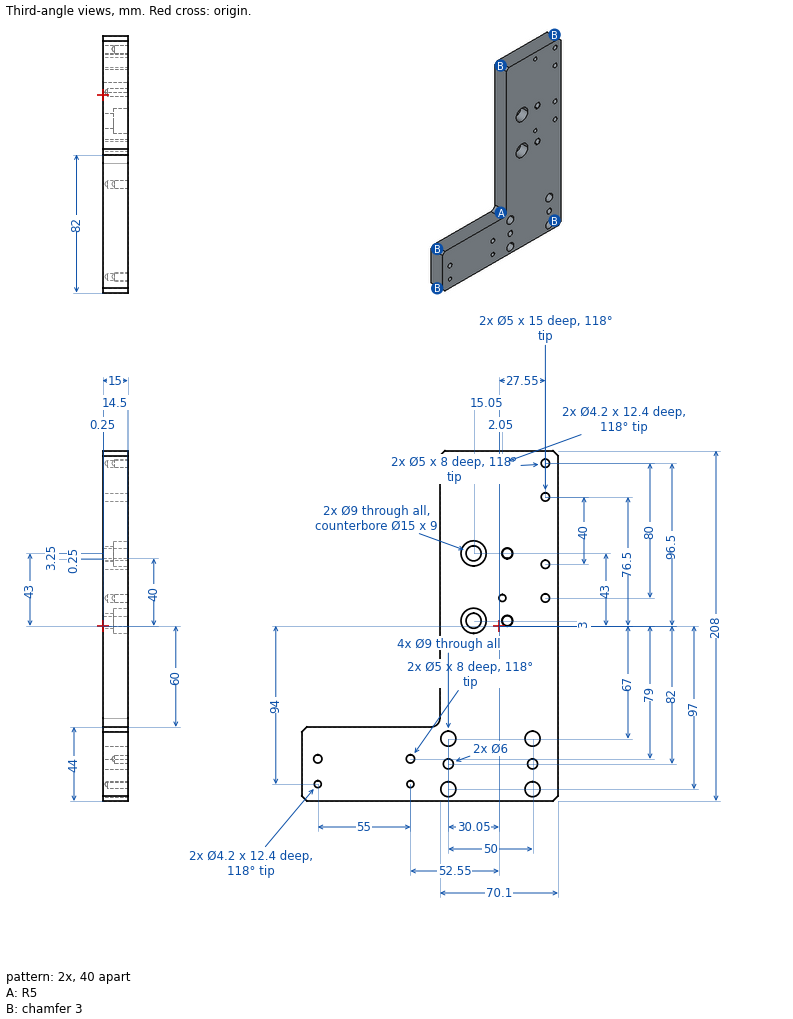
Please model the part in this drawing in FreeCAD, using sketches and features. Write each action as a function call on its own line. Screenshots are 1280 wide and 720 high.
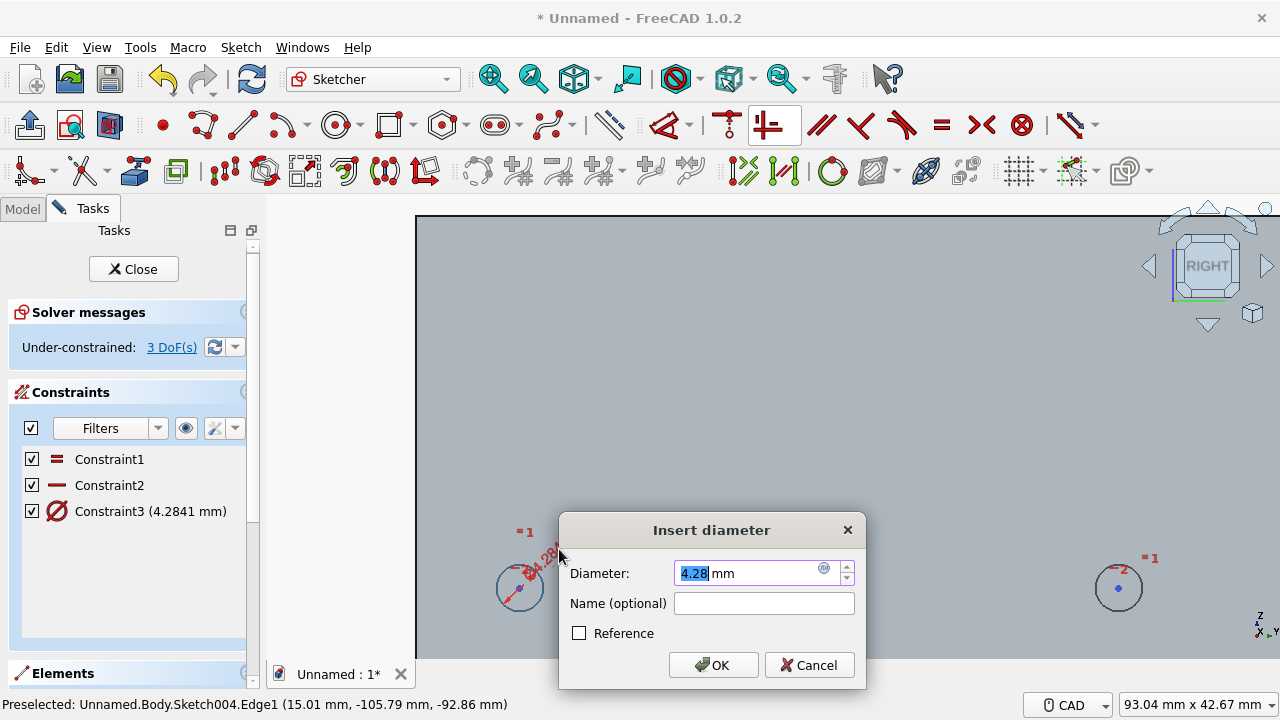
text(4.2)
key(Return)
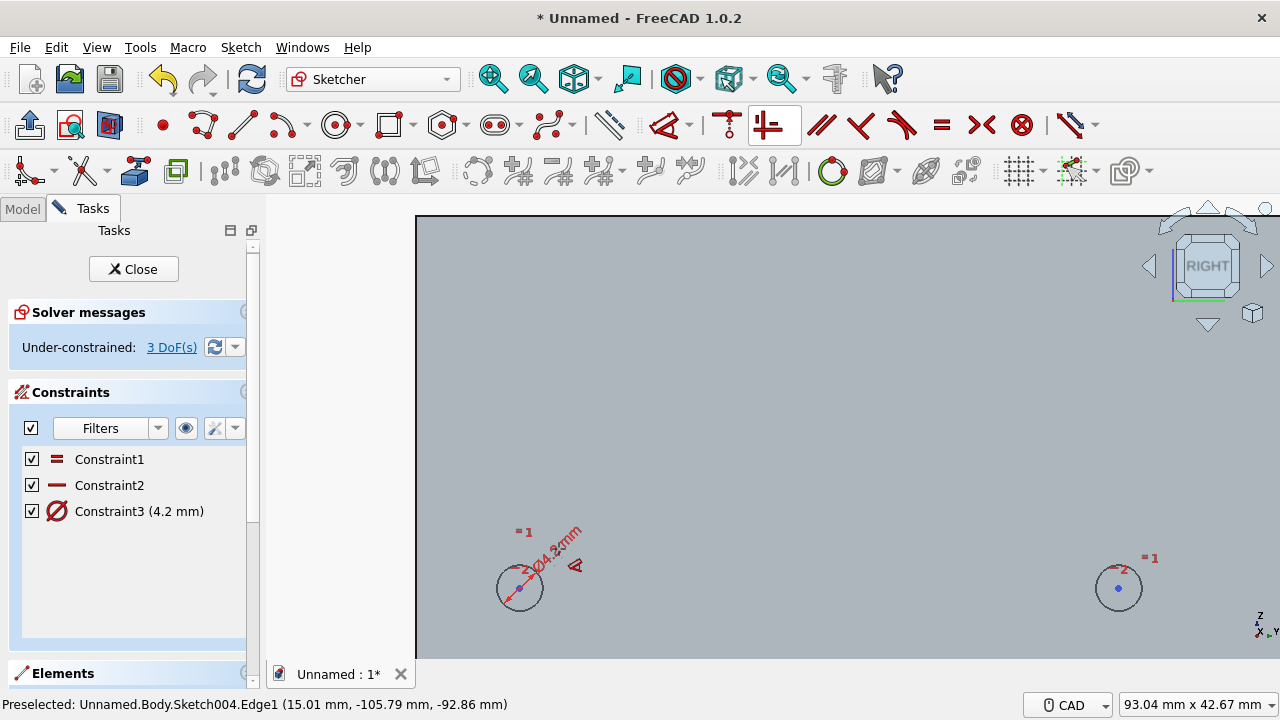
click(520, 588)
click(486, 405)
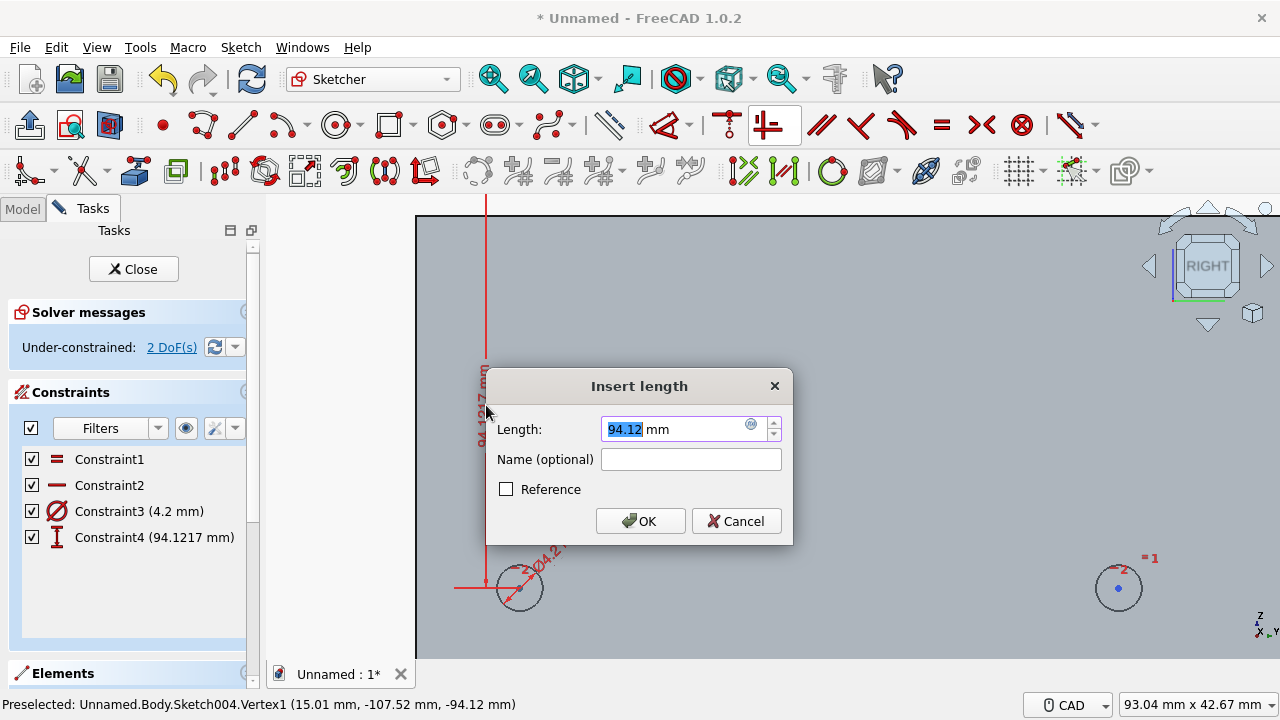
text(94)
key(Return)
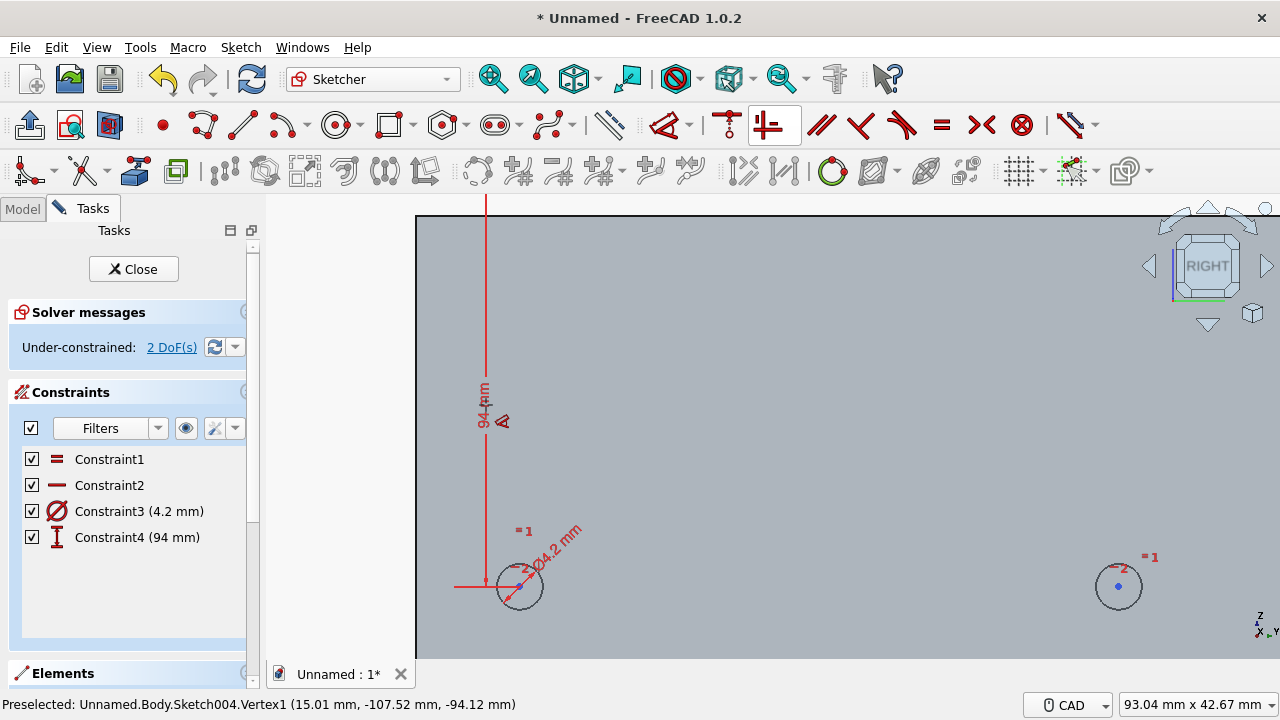
click(520, 587)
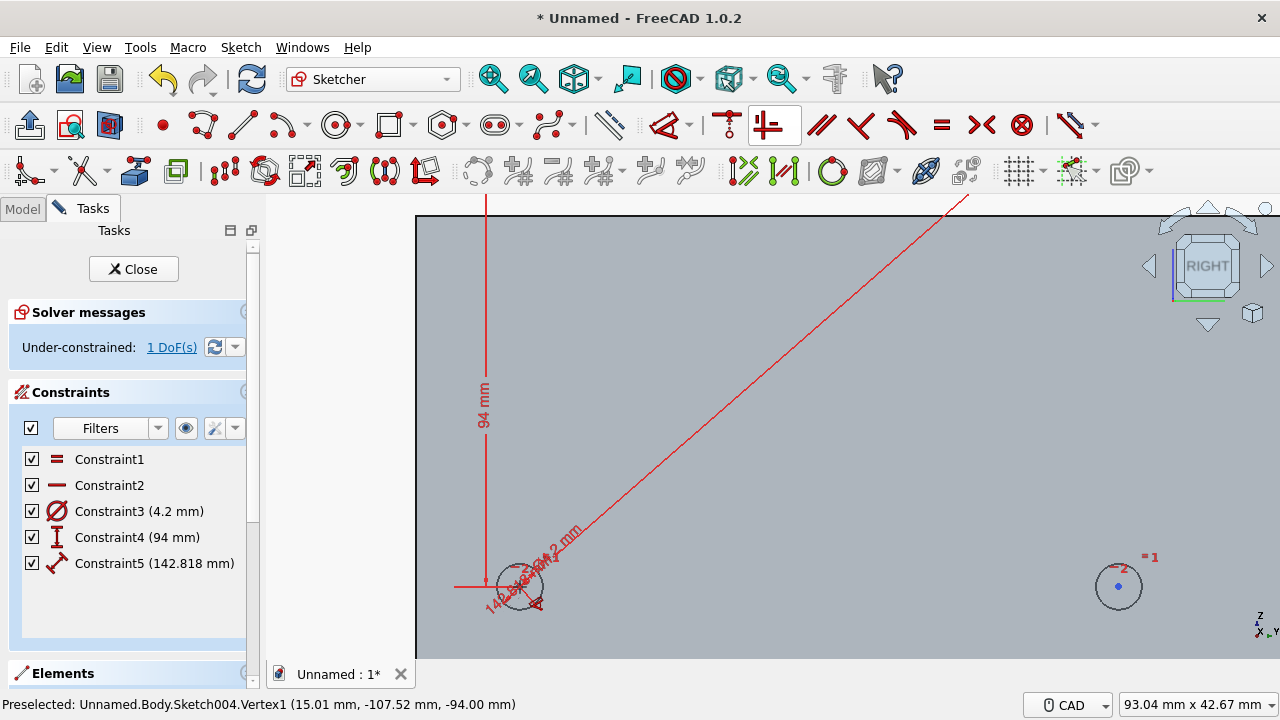
scroll(537, 573, down, 6)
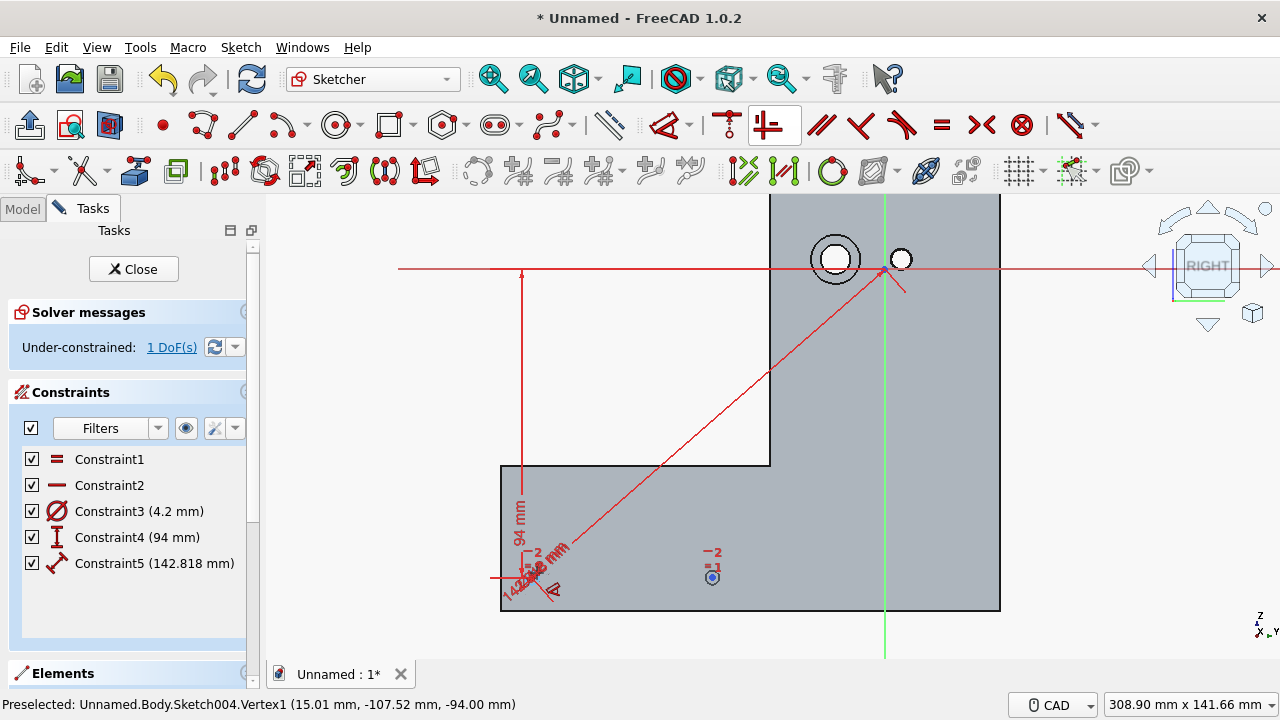
click(712, 578)
click(622, 612)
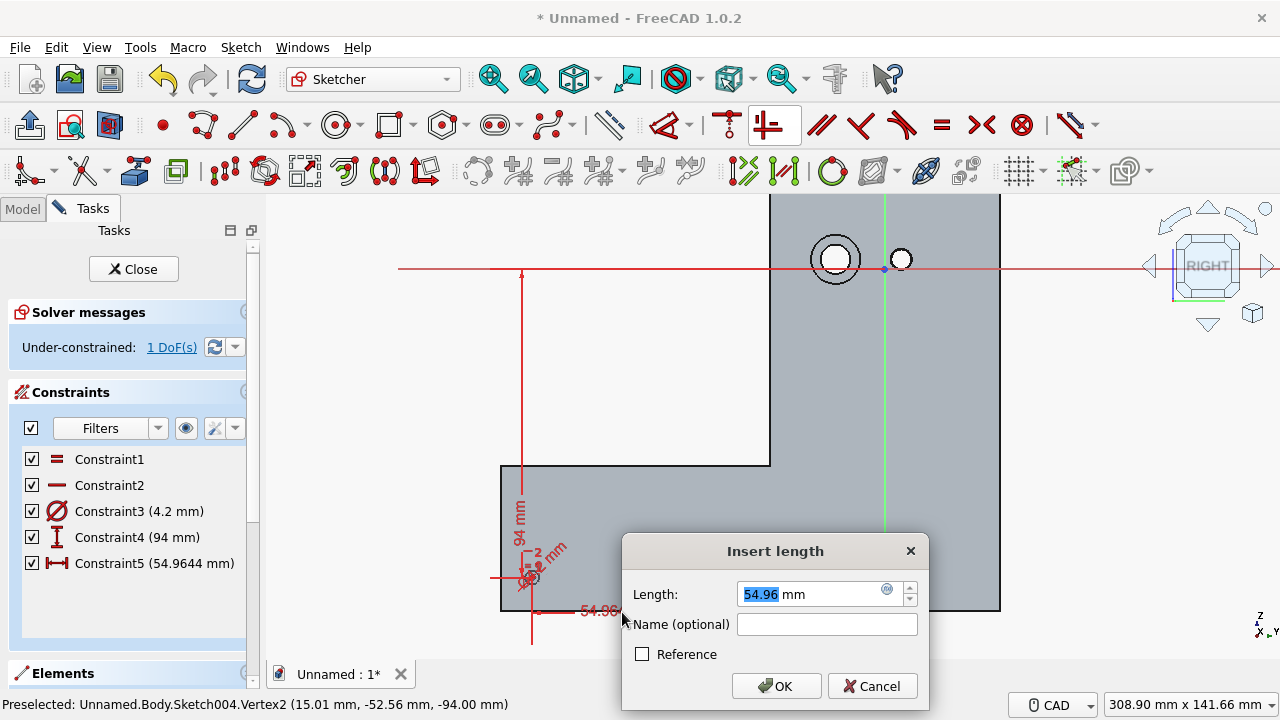
text(55)
key(Return)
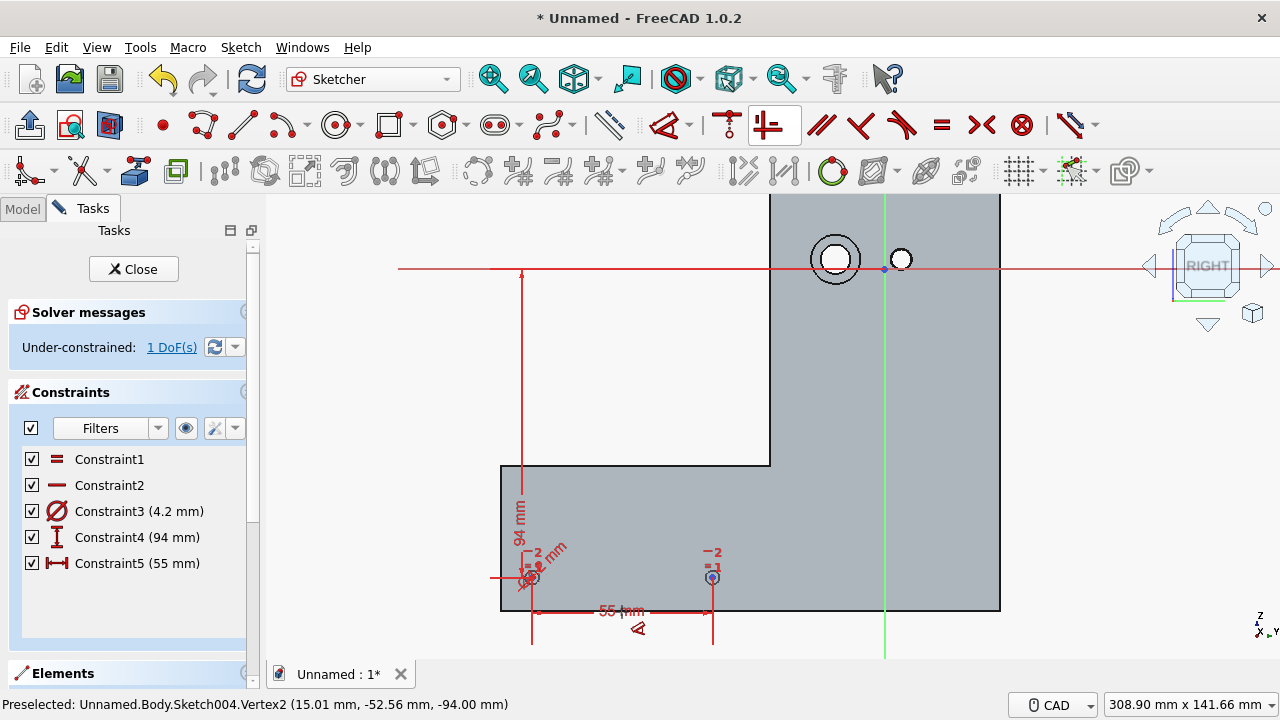
click(713, 578)
click(799, 235)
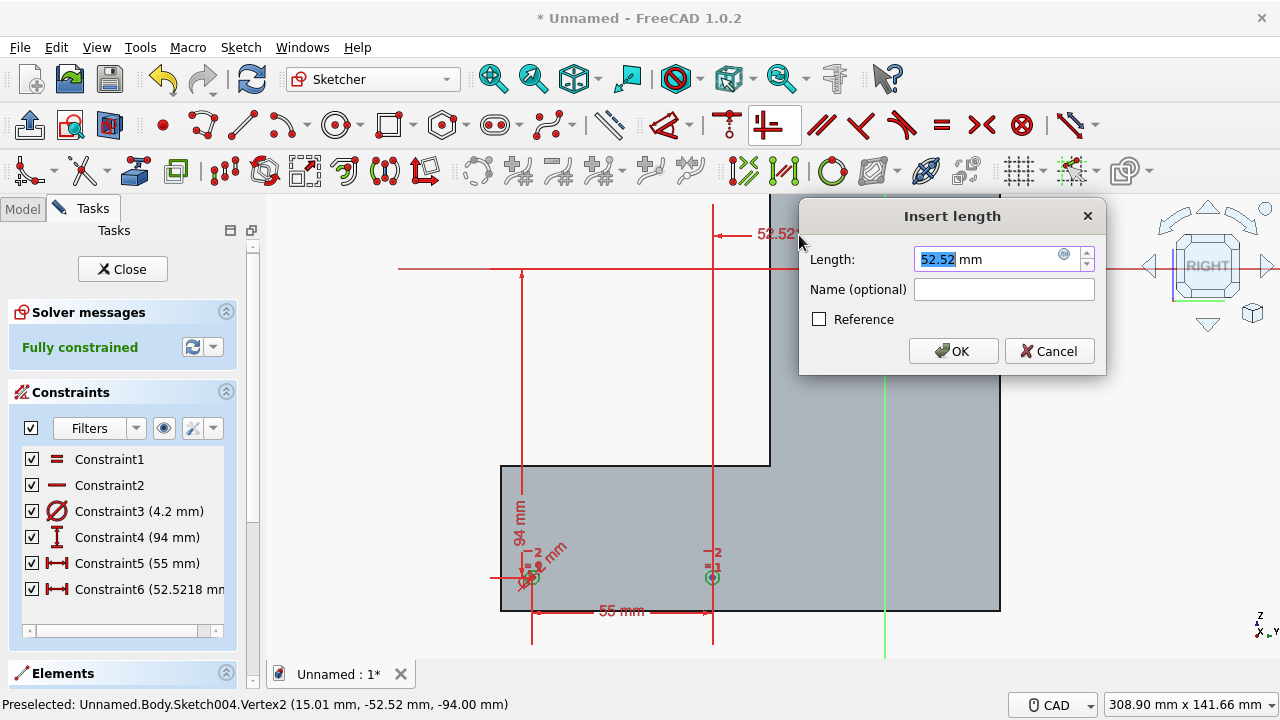
text(52.55)
key(Return)
key(Escape)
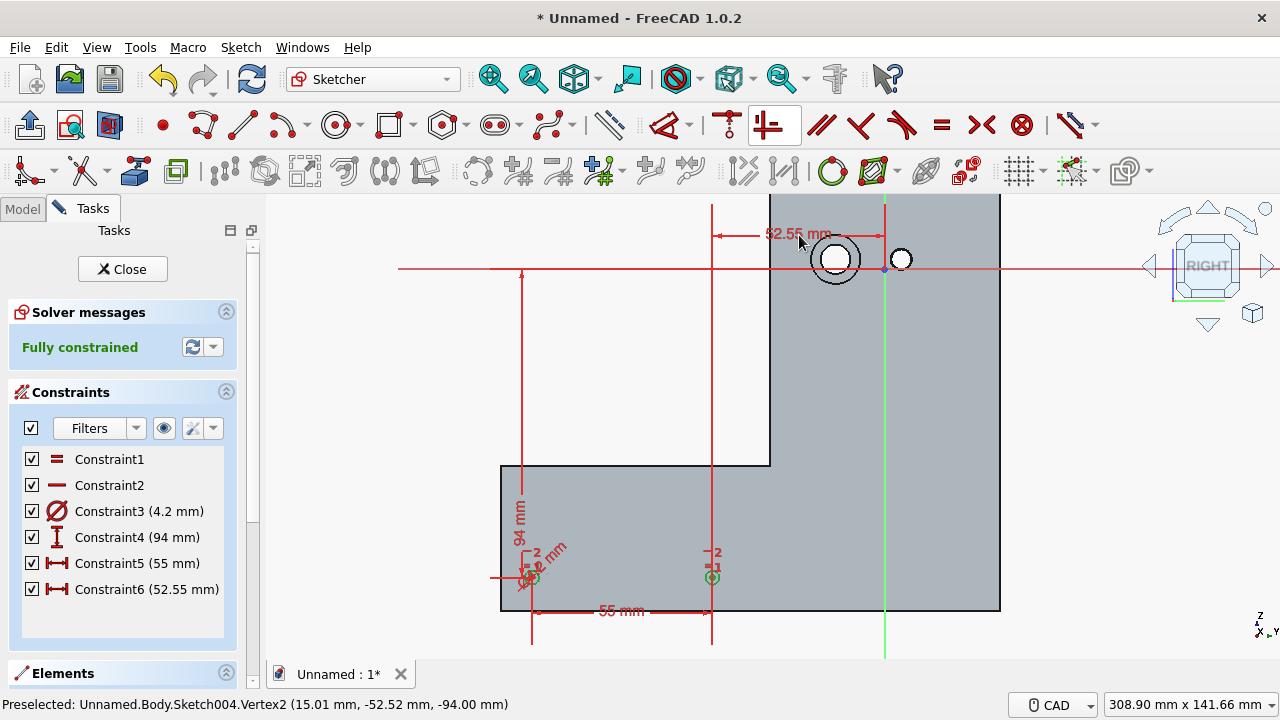
click(123, 269)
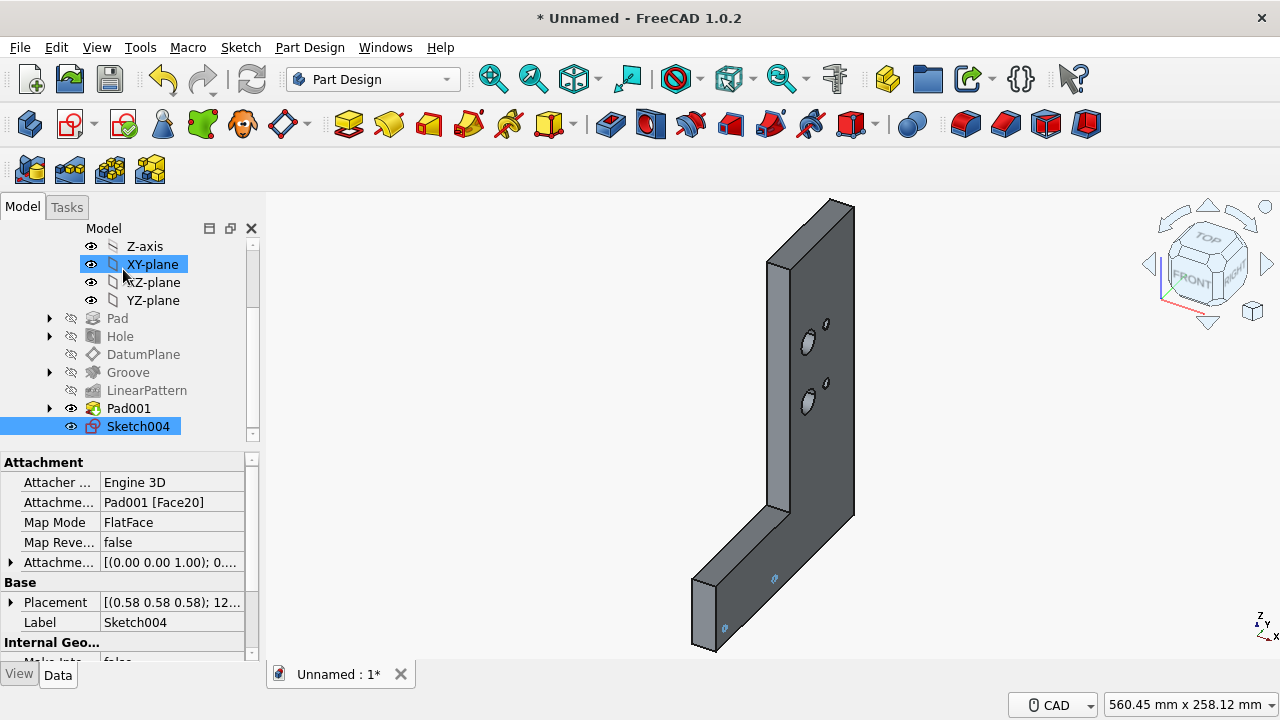
click(652, 124)